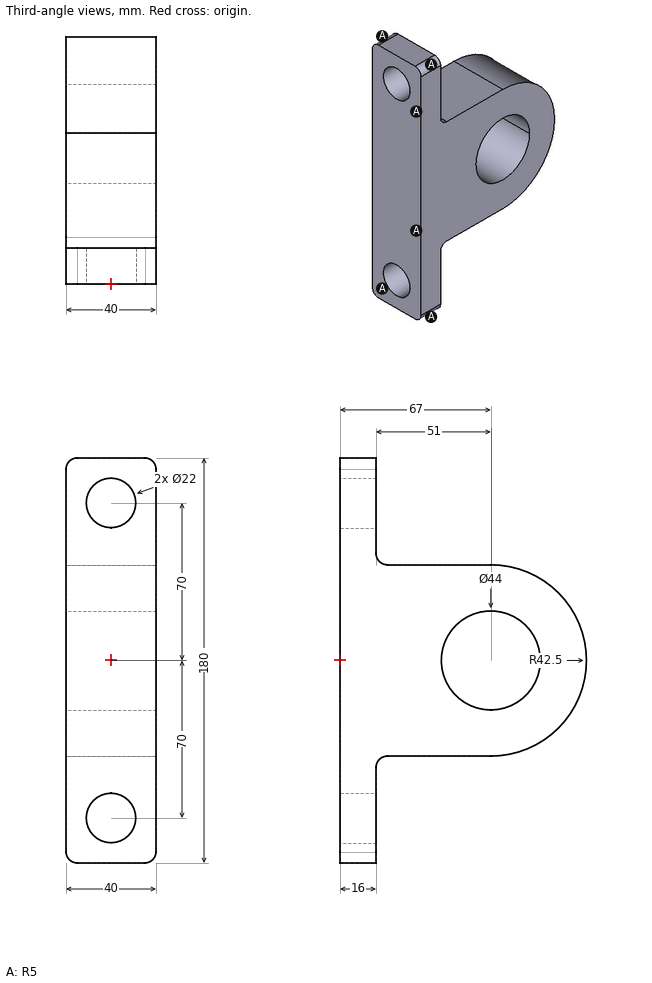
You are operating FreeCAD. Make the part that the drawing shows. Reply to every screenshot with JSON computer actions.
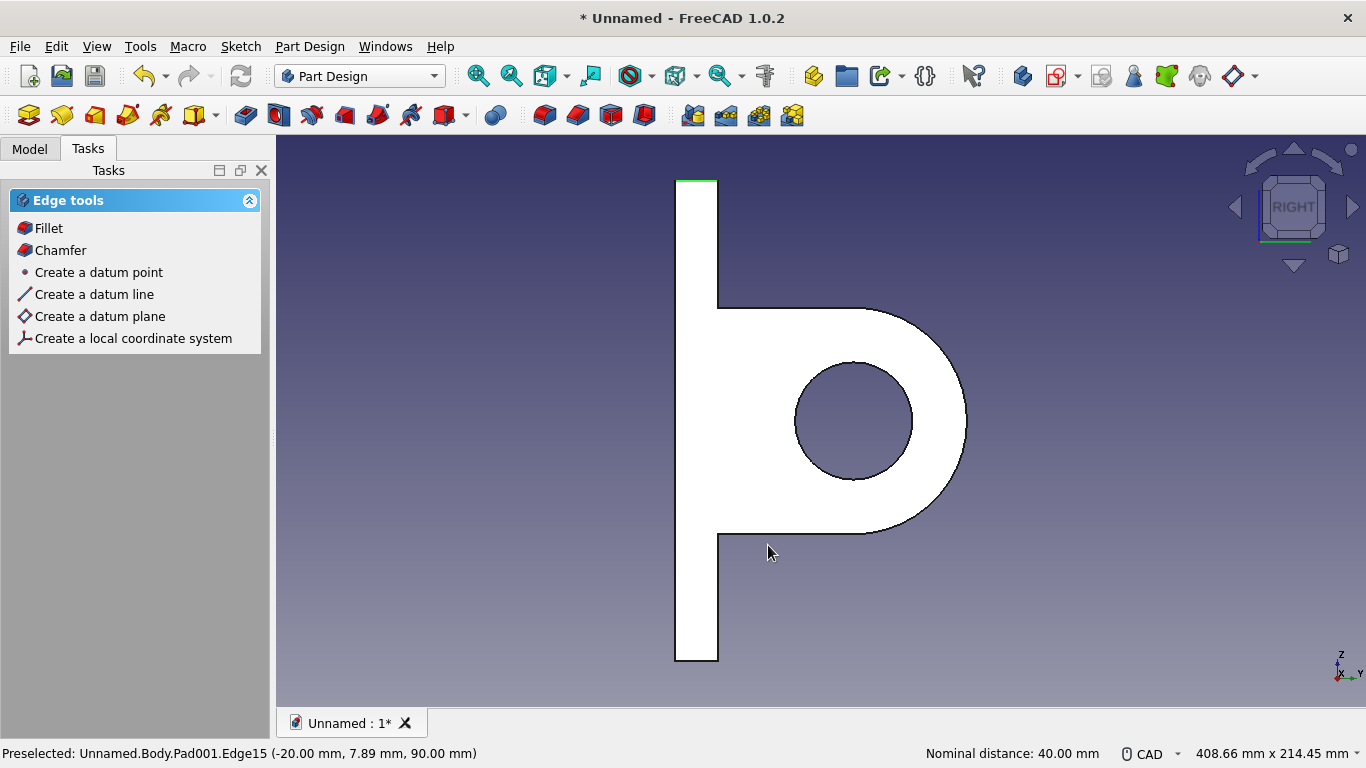
{"action": "left_click", "coordinate": [696, 660], "text": "ctrl"}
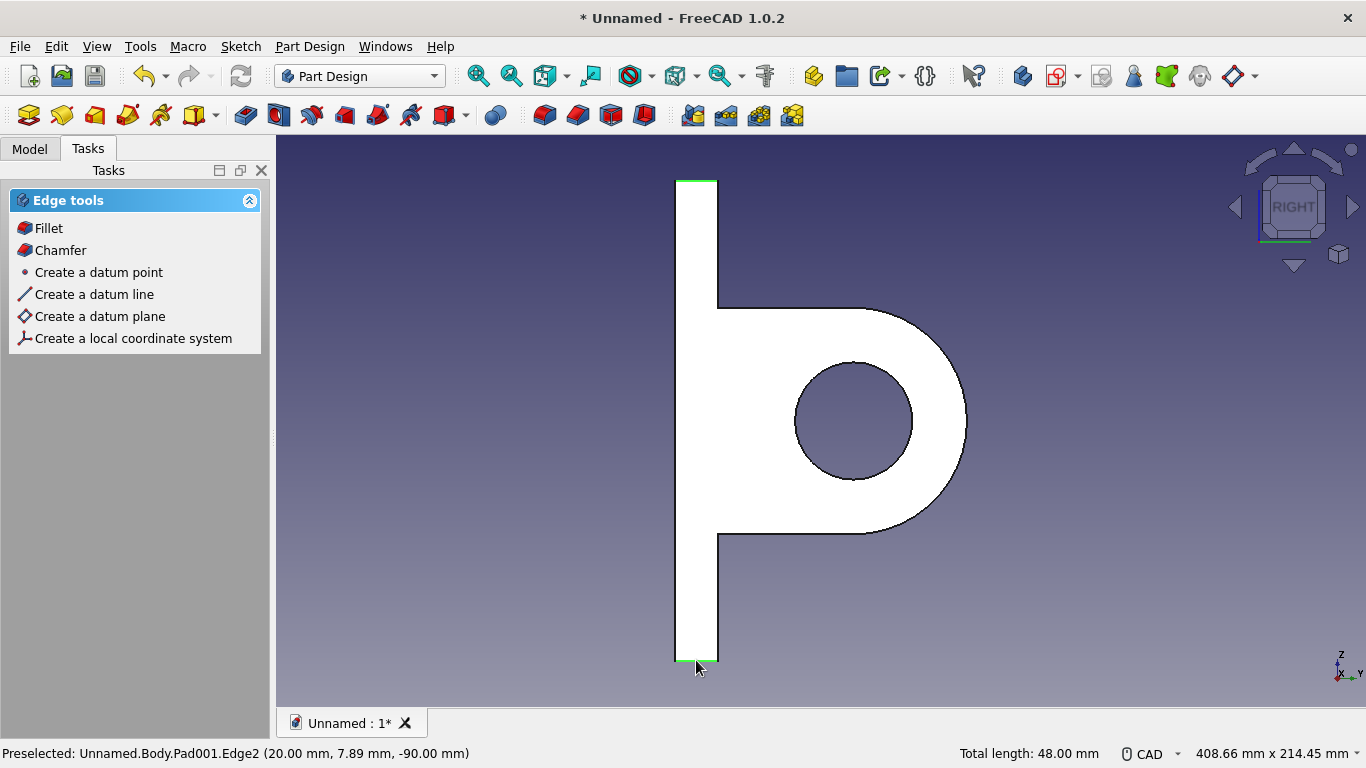
{"action": "key", "text": "5"}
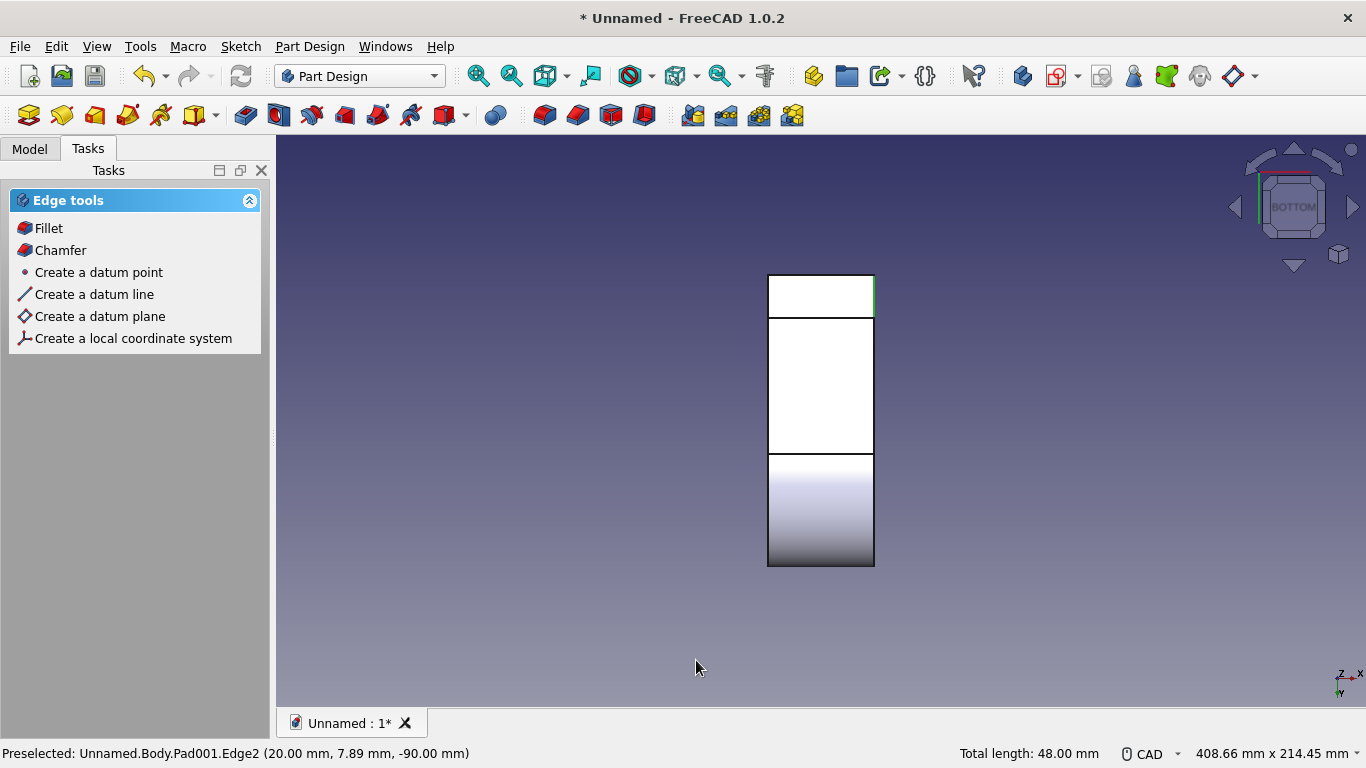
{"action": "left_click", "coordinate": [768, 295], "text": "ctrl"}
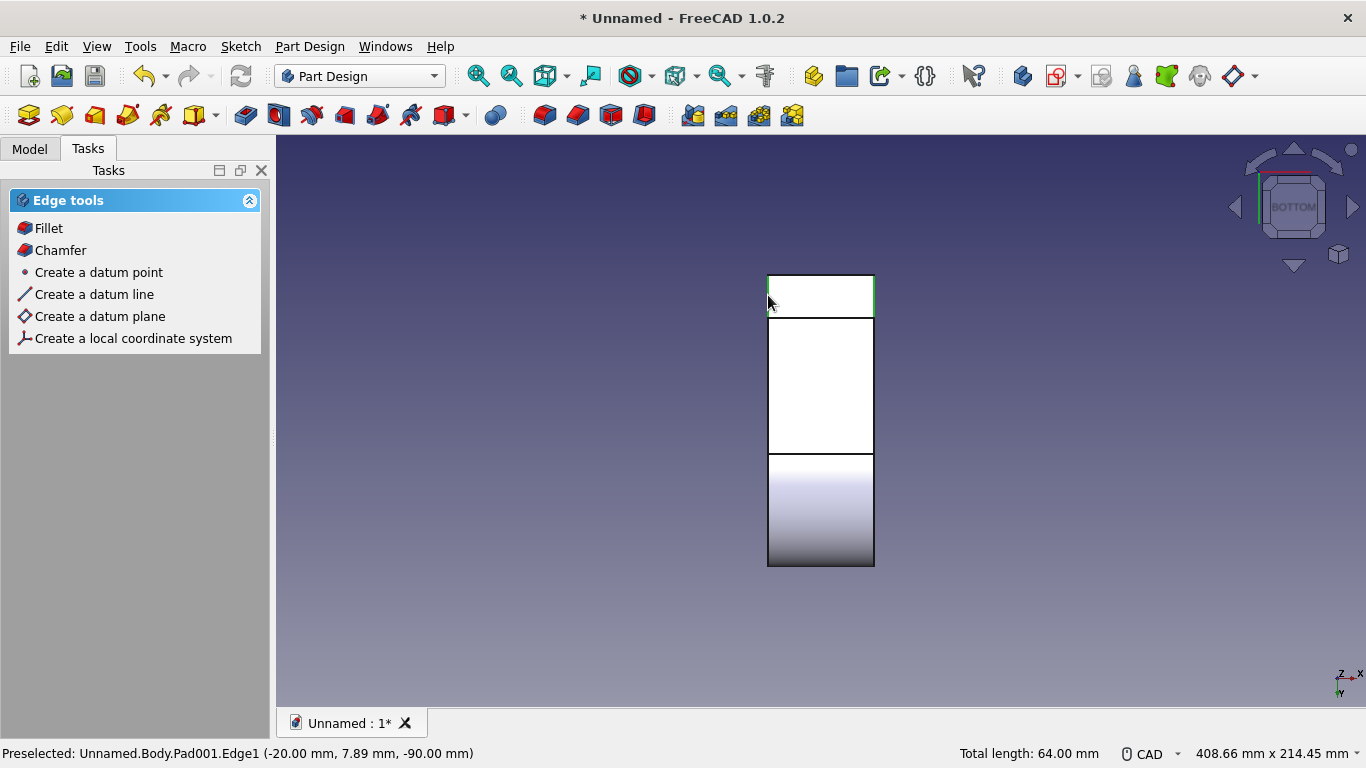
{"action": "key", "text": "4"}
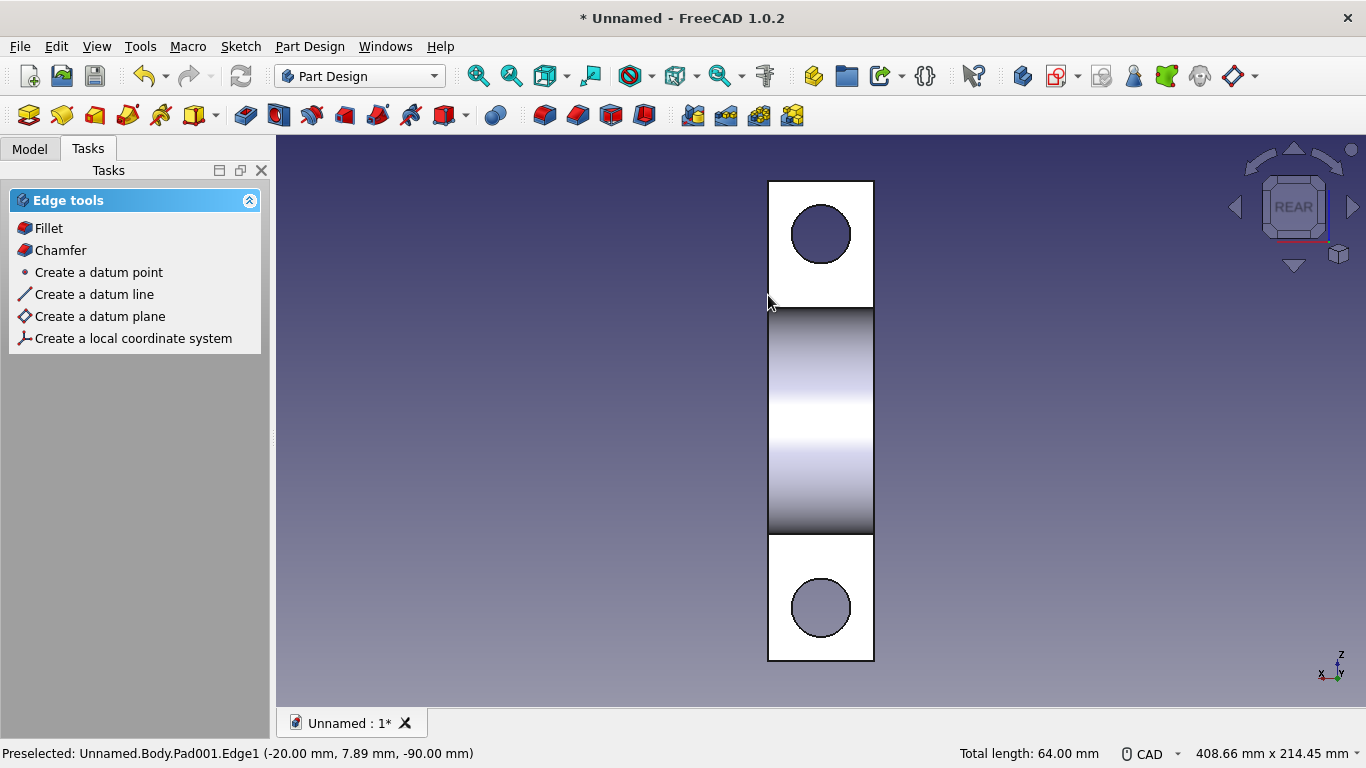
{"action": "key", "text": "6"}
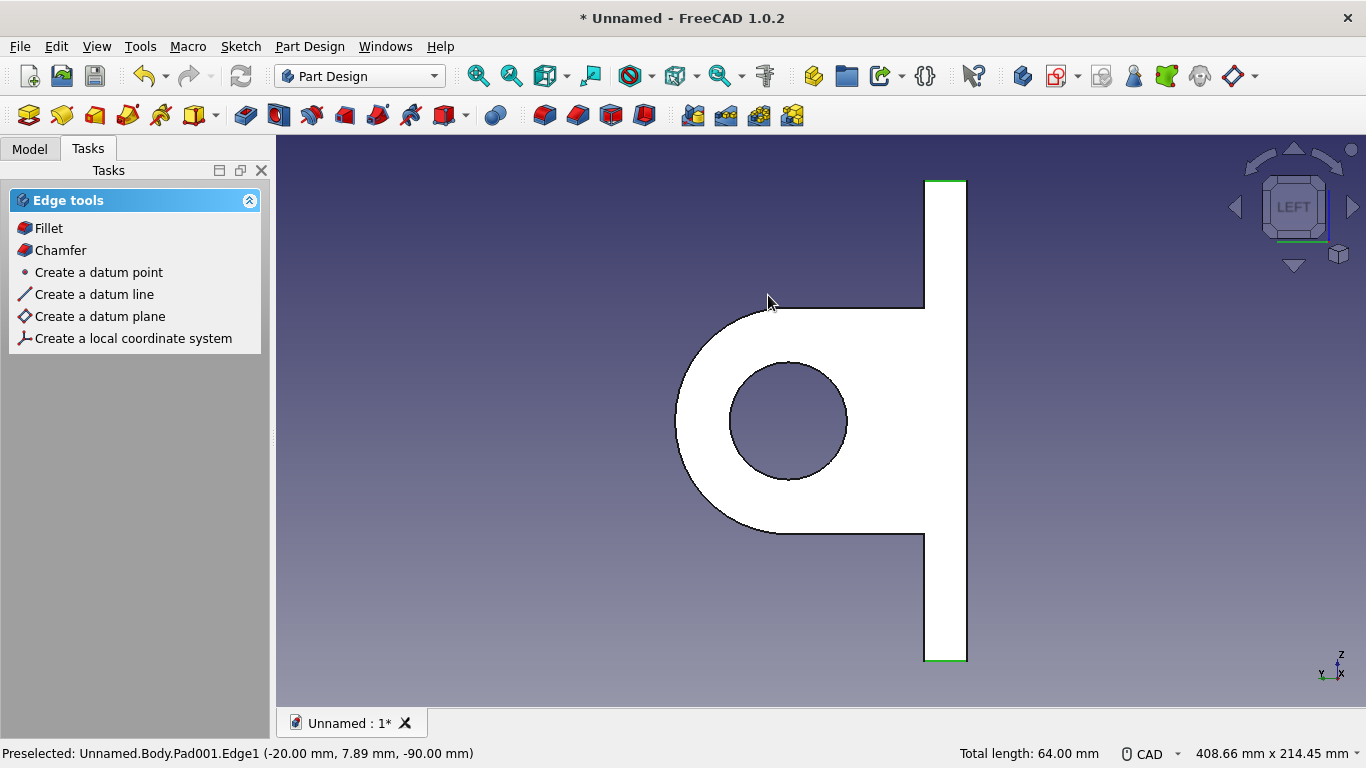
{"action": "key", "text": "v 3"}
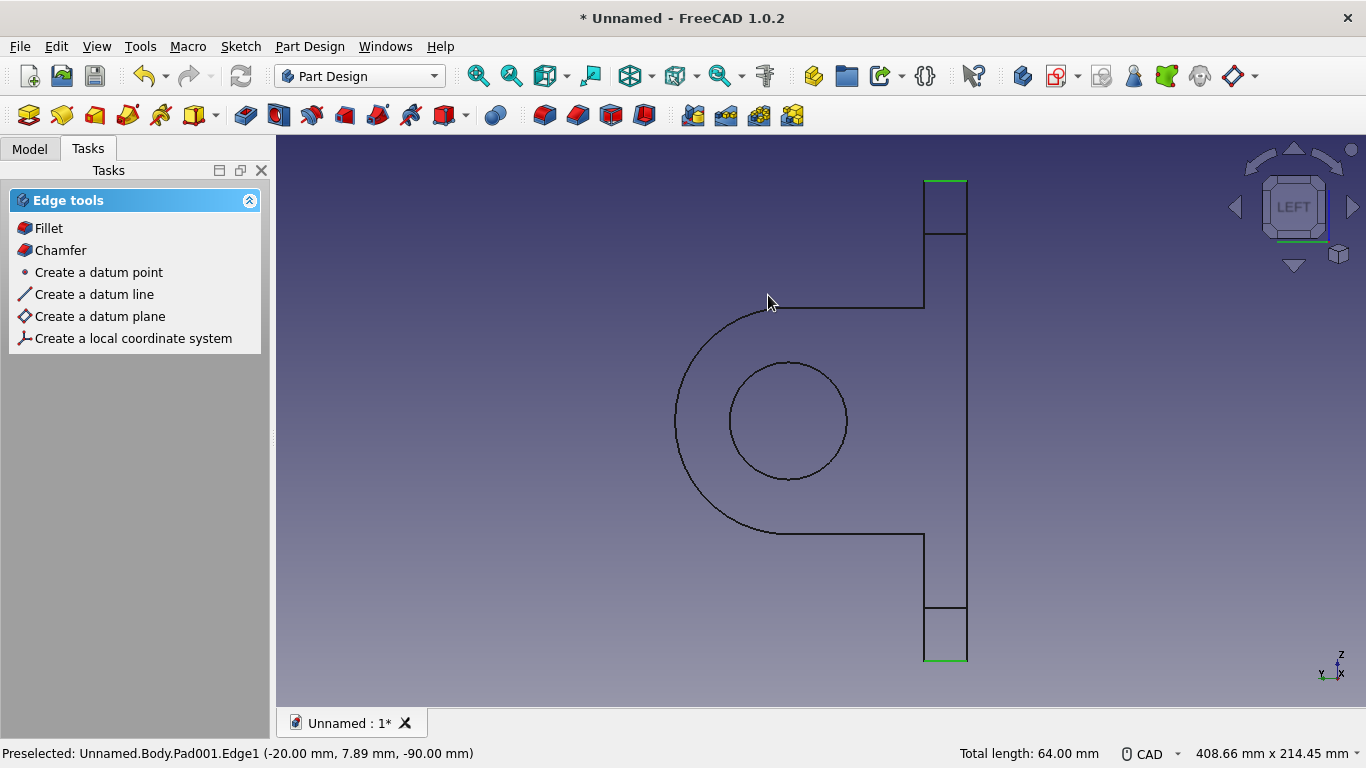
{"action": "key", "text": "0"}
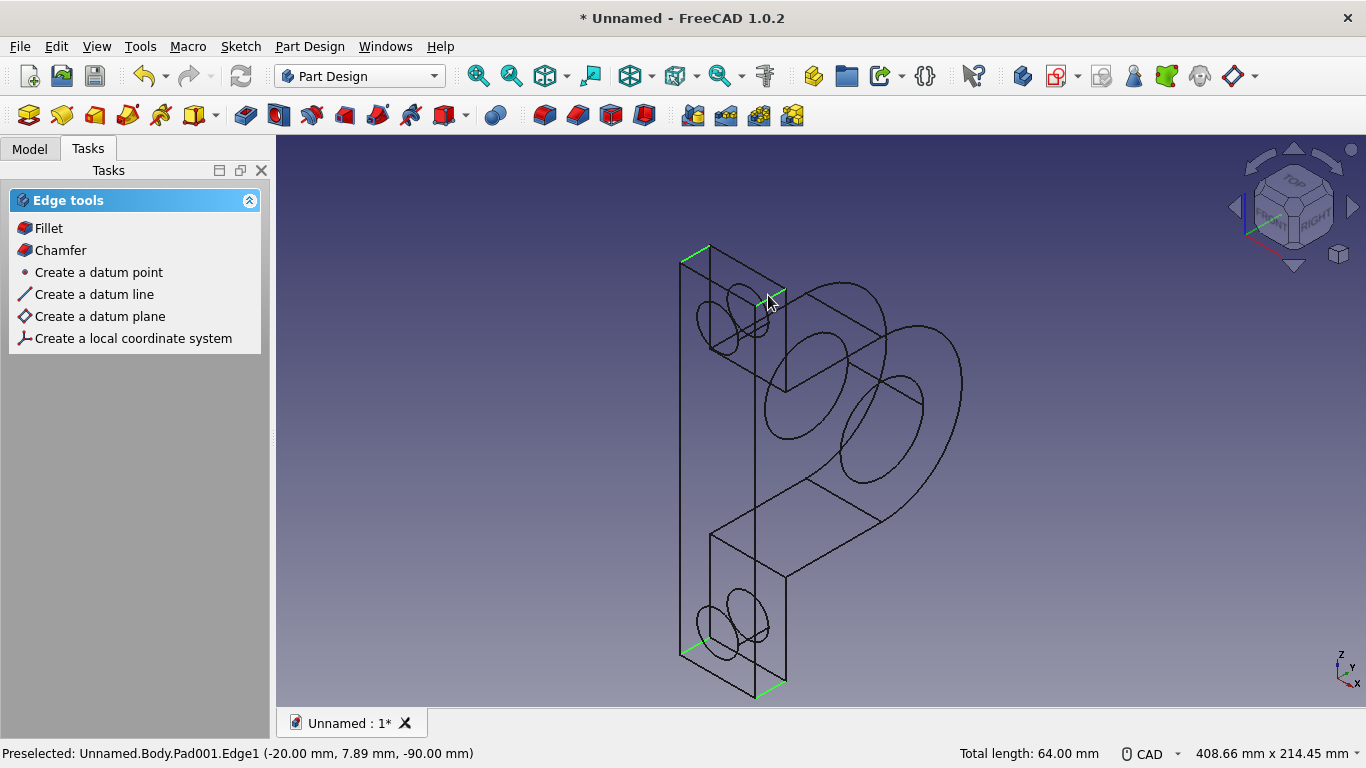
{"action": "left_click", "coordinate": [748, 370], "text": "ctrl"}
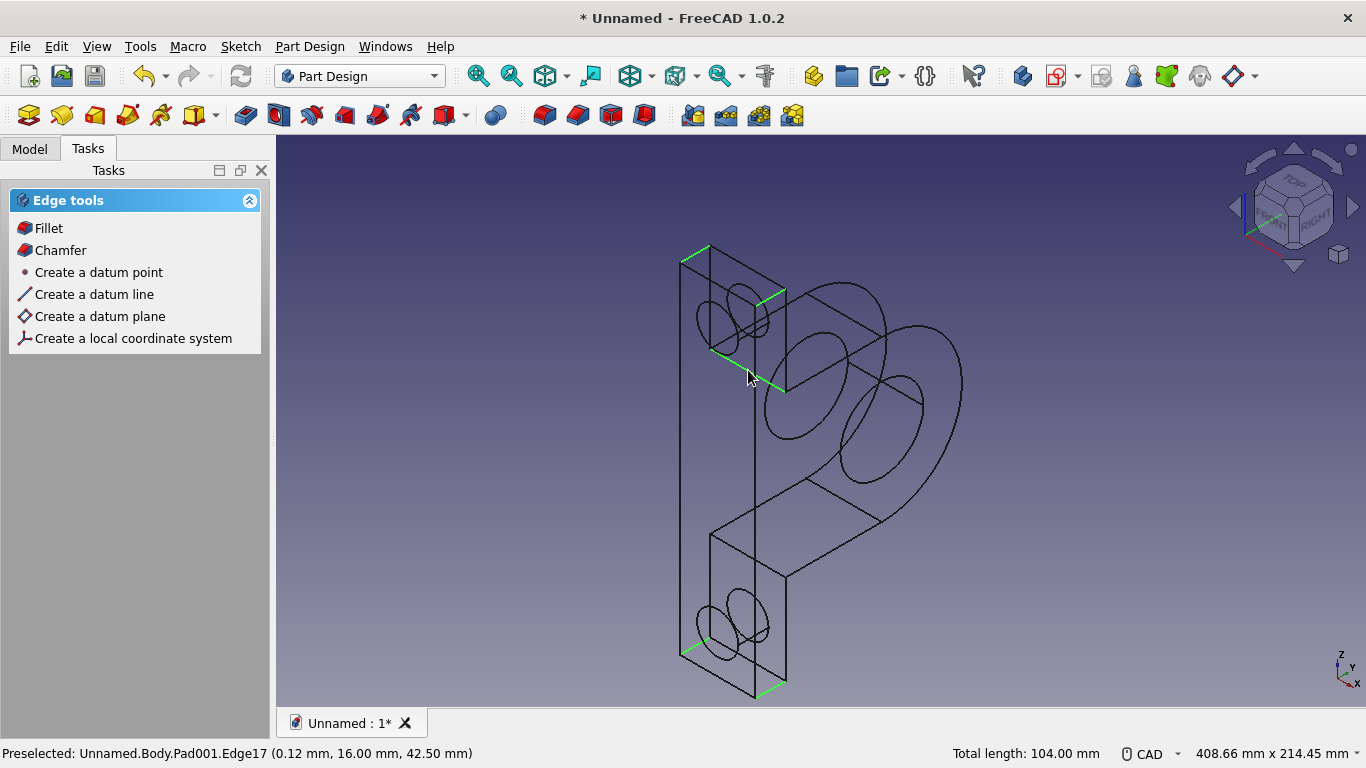
{"action": "left_click", "coordinate": [748, 555], "text": "ctrl"}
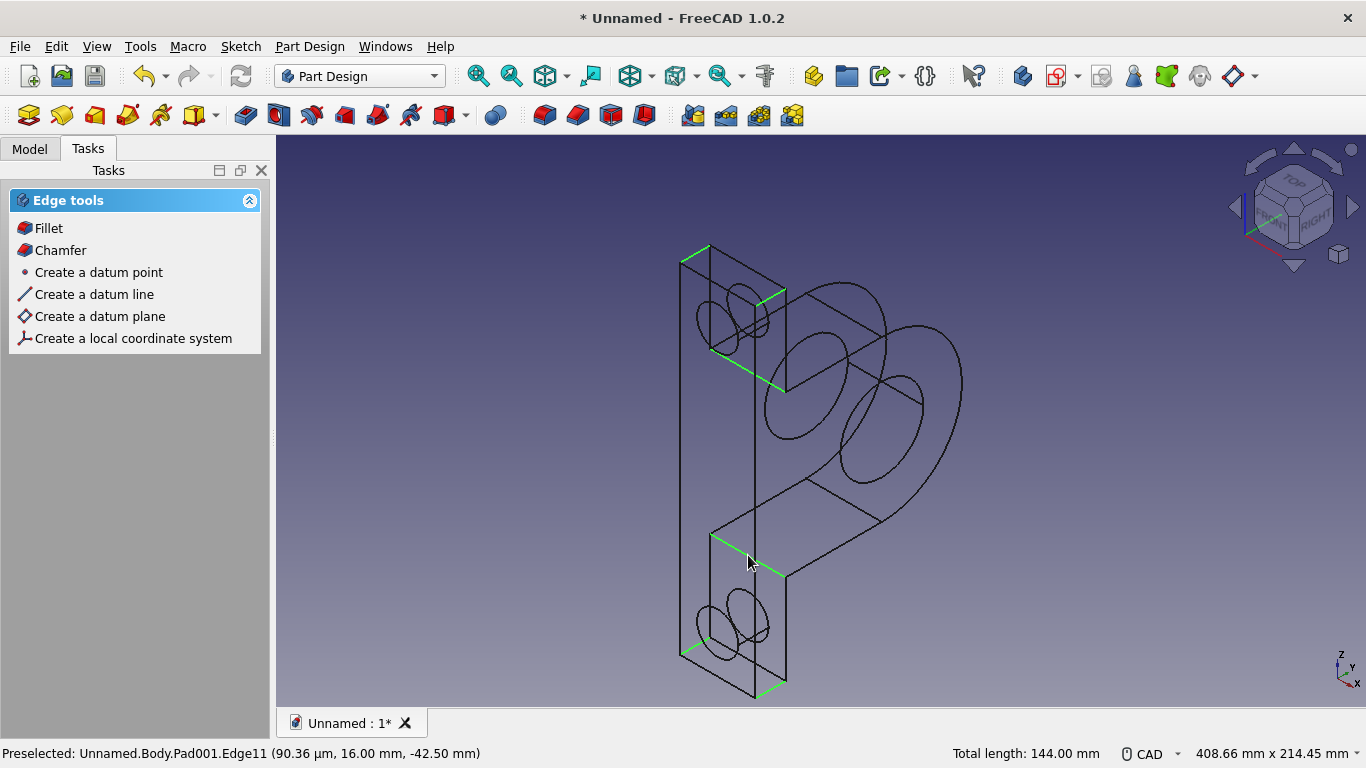
{"action": "key", "text": "v 1"}